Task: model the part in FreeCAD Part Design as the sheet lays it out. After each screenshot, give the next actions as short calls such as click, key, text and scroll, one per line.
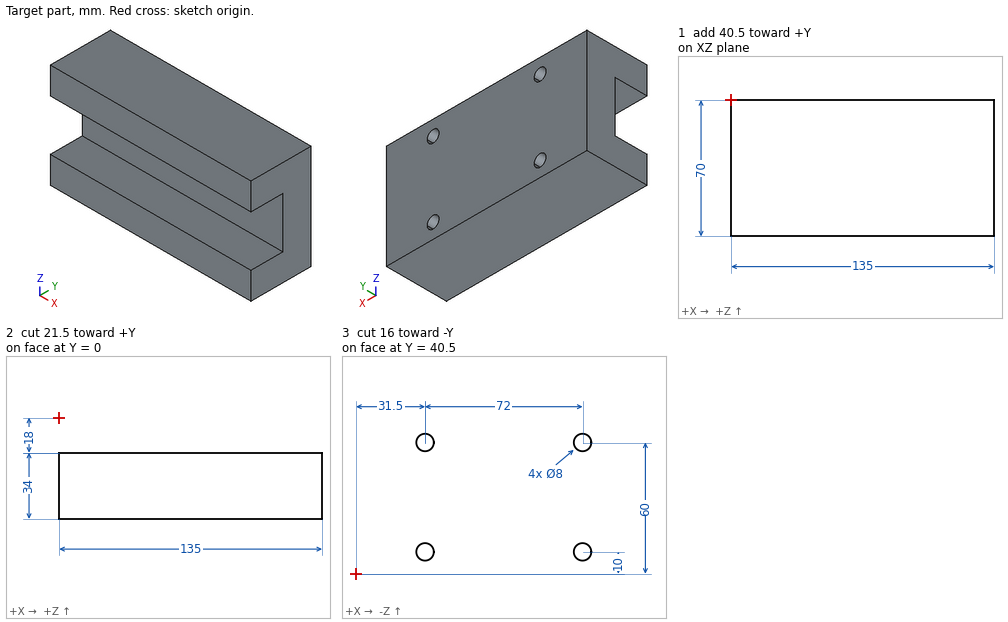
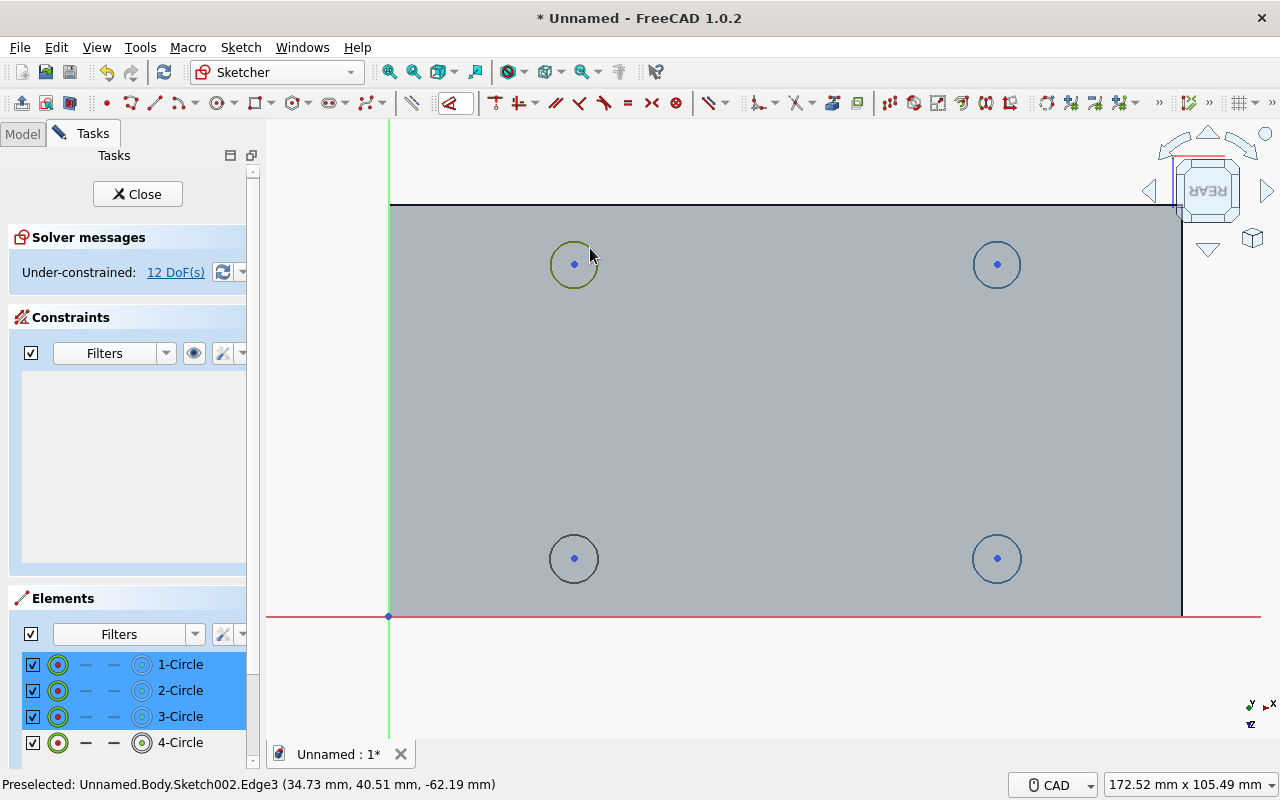
click(591, 542)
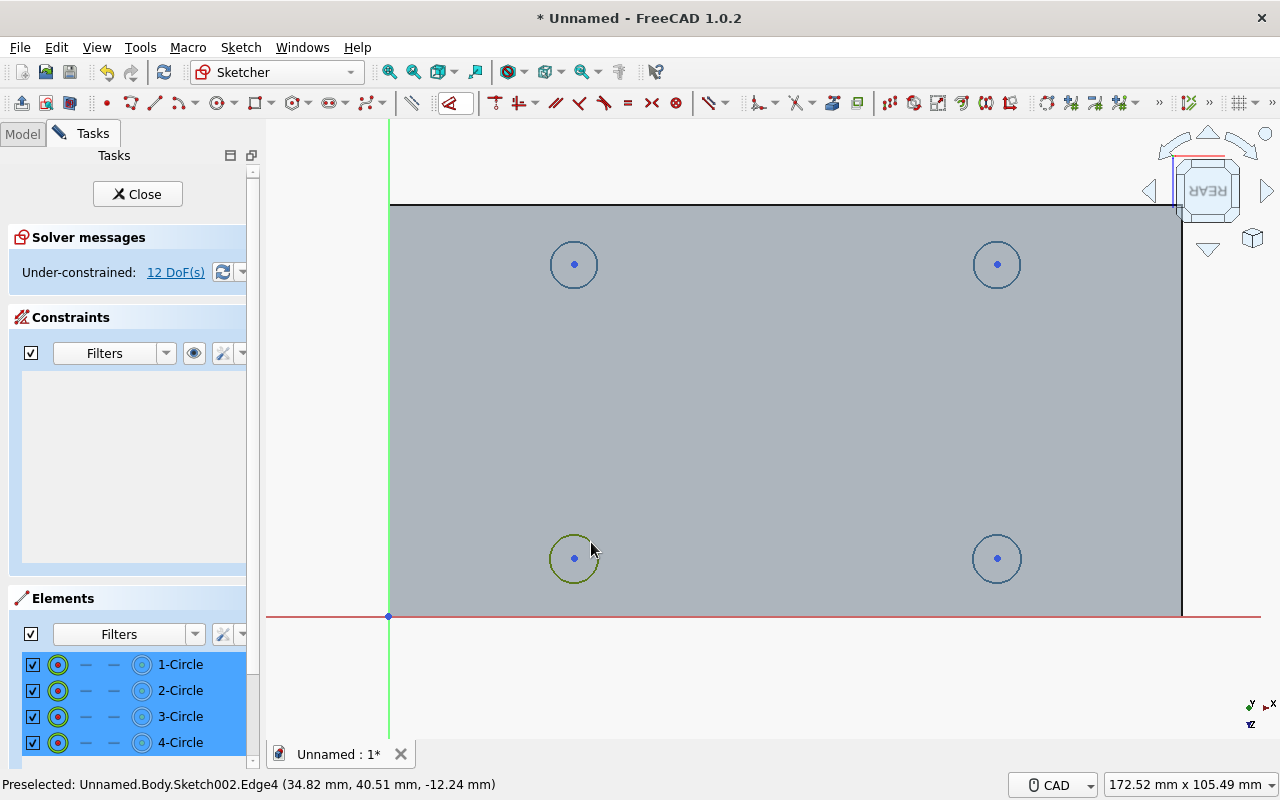
click(628, 104)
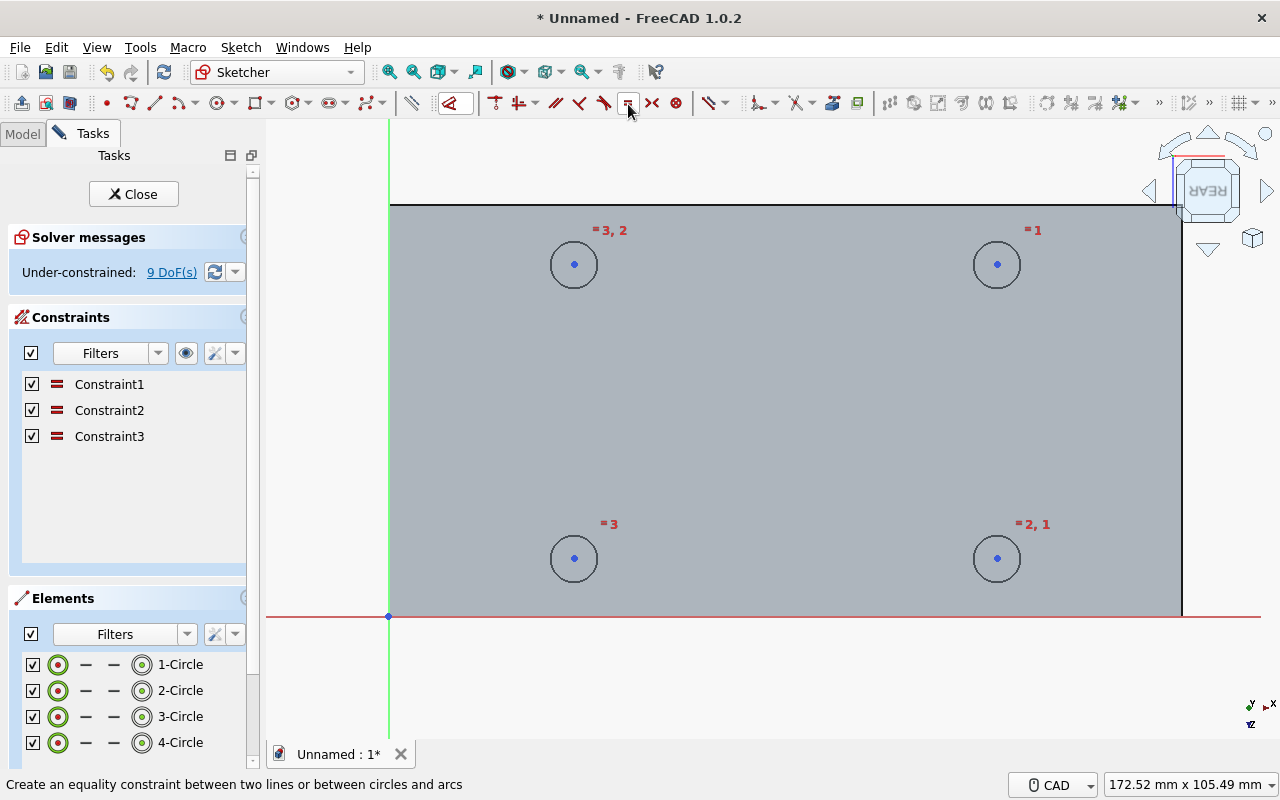
click(997, 265)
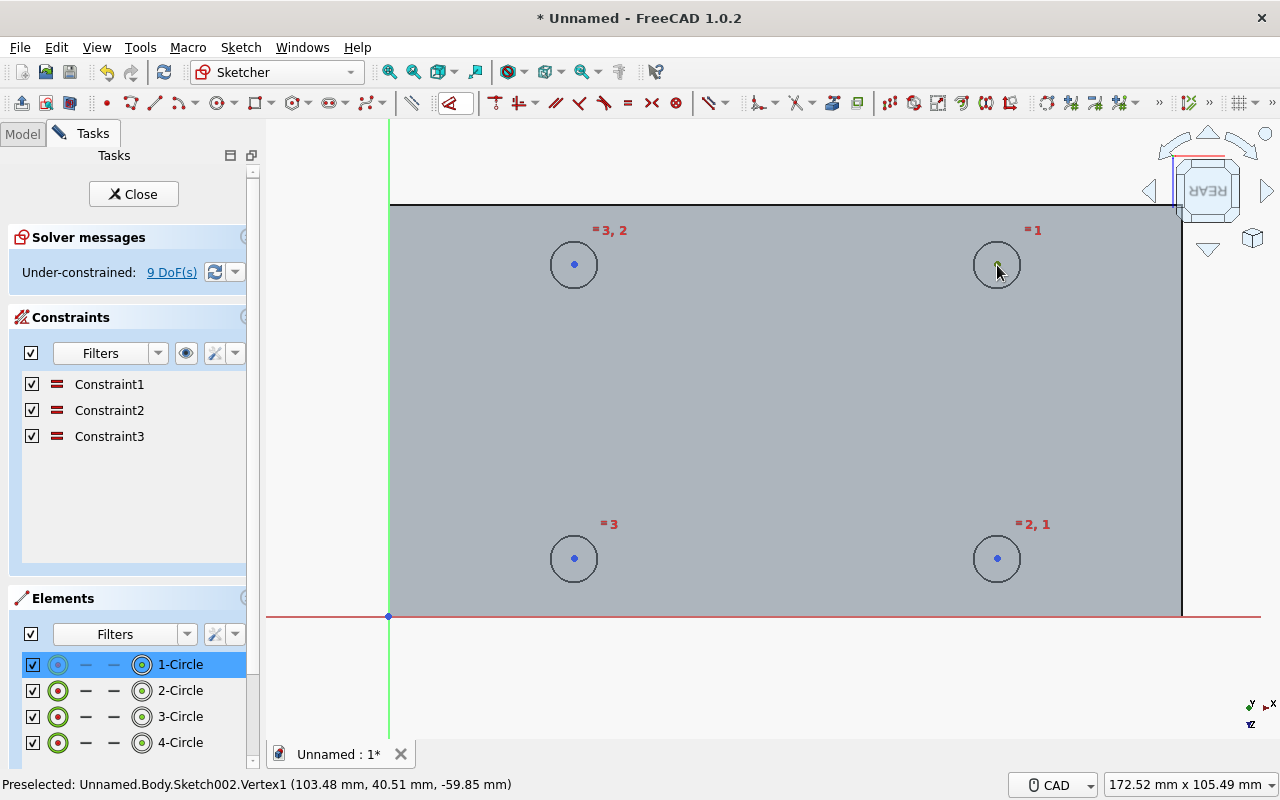
click(997, 559)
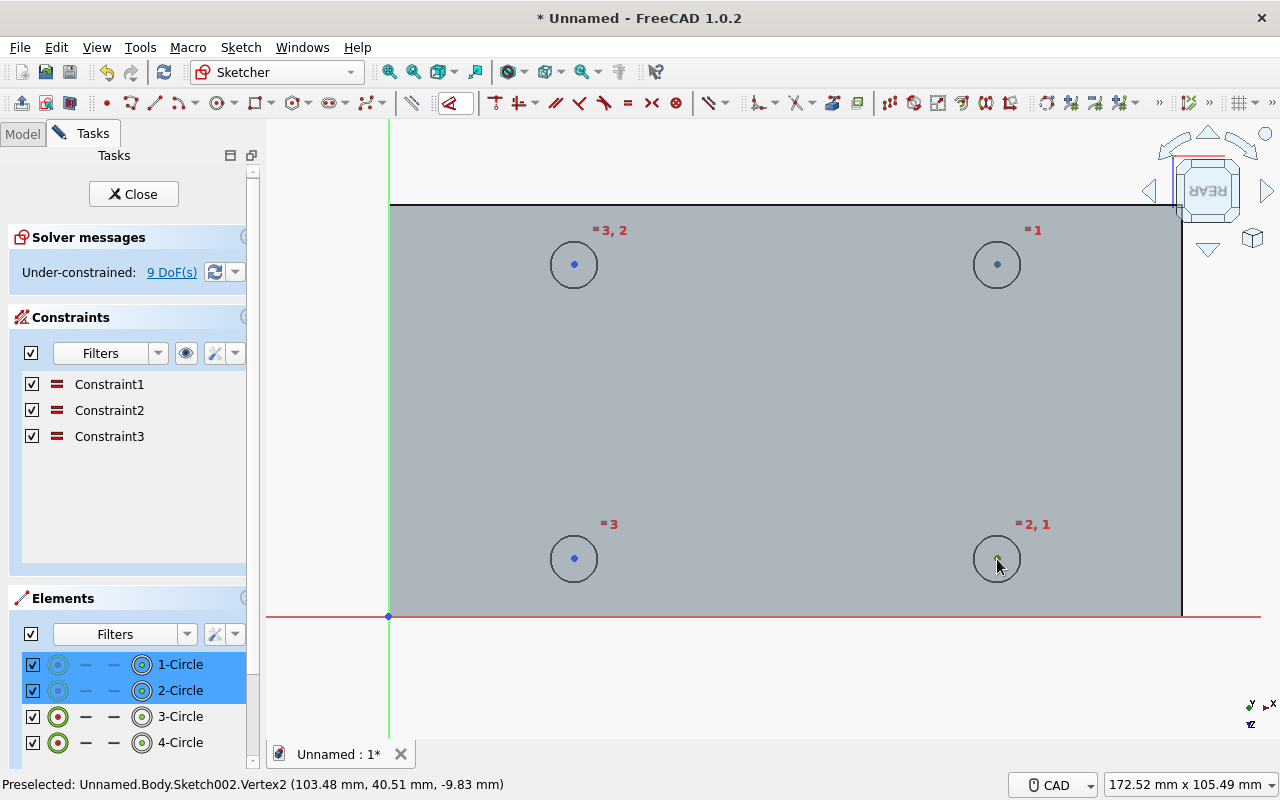
click(538, 104)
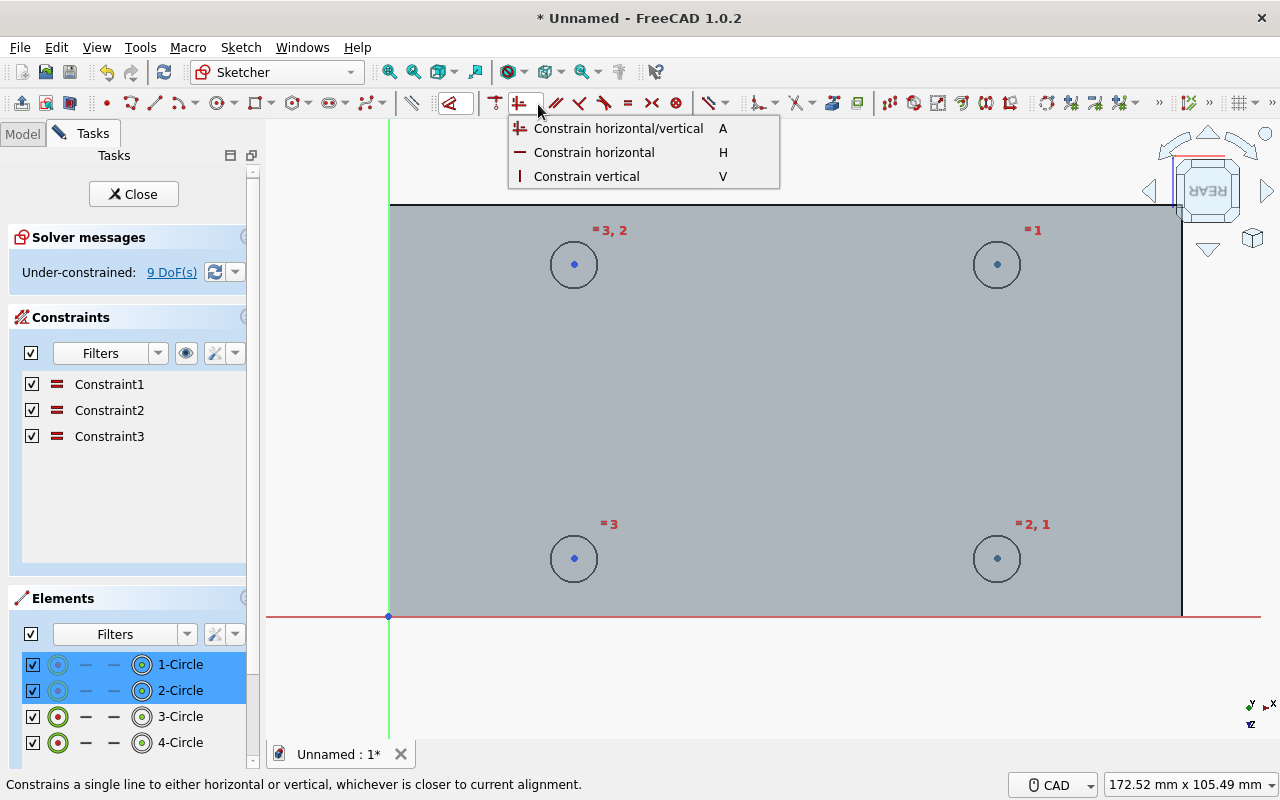
click(644, 176)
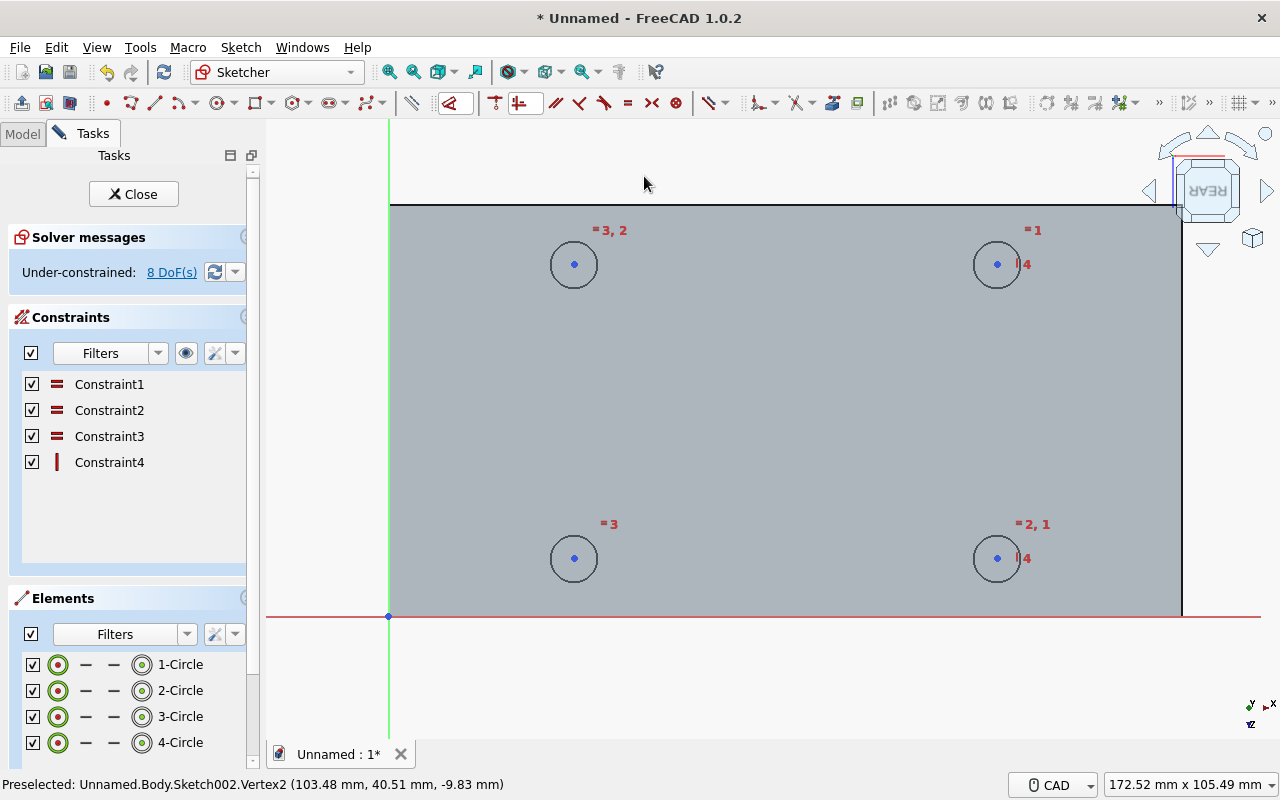
click(997, 265)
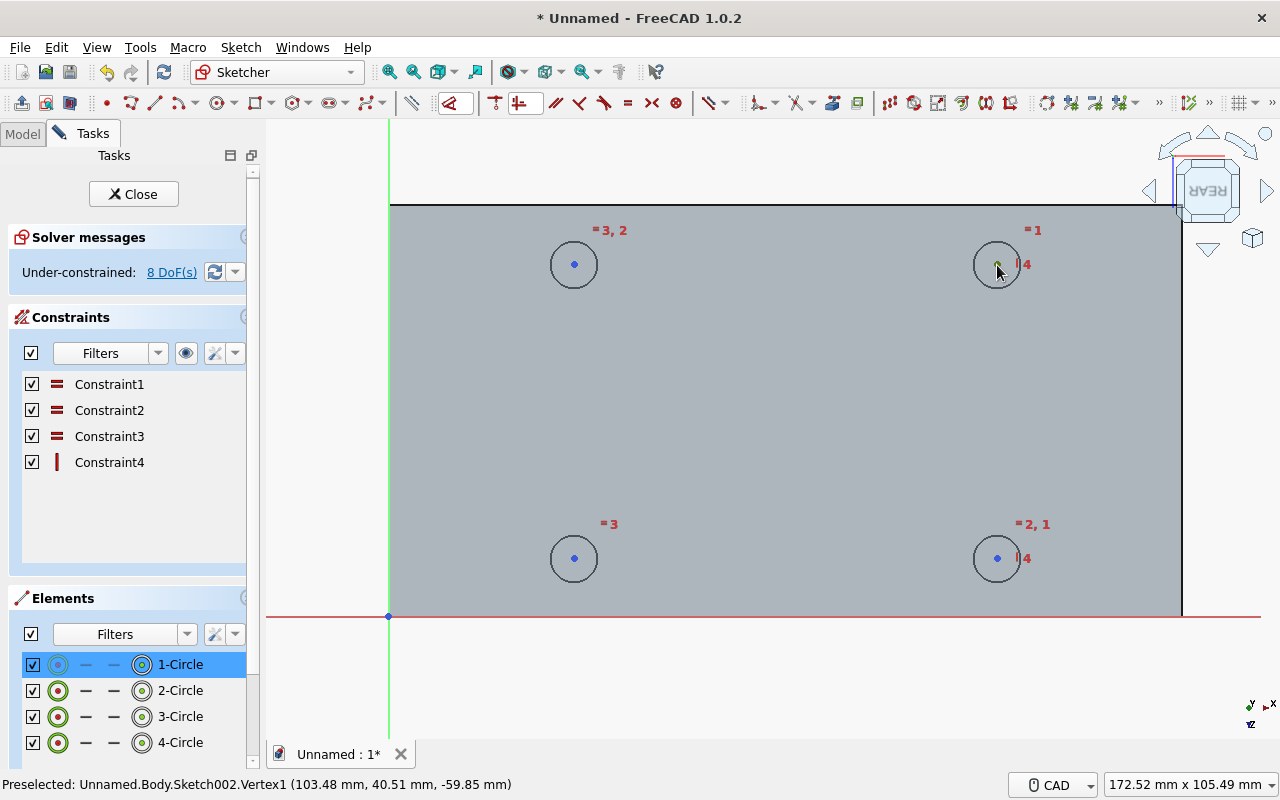
click(574, 265)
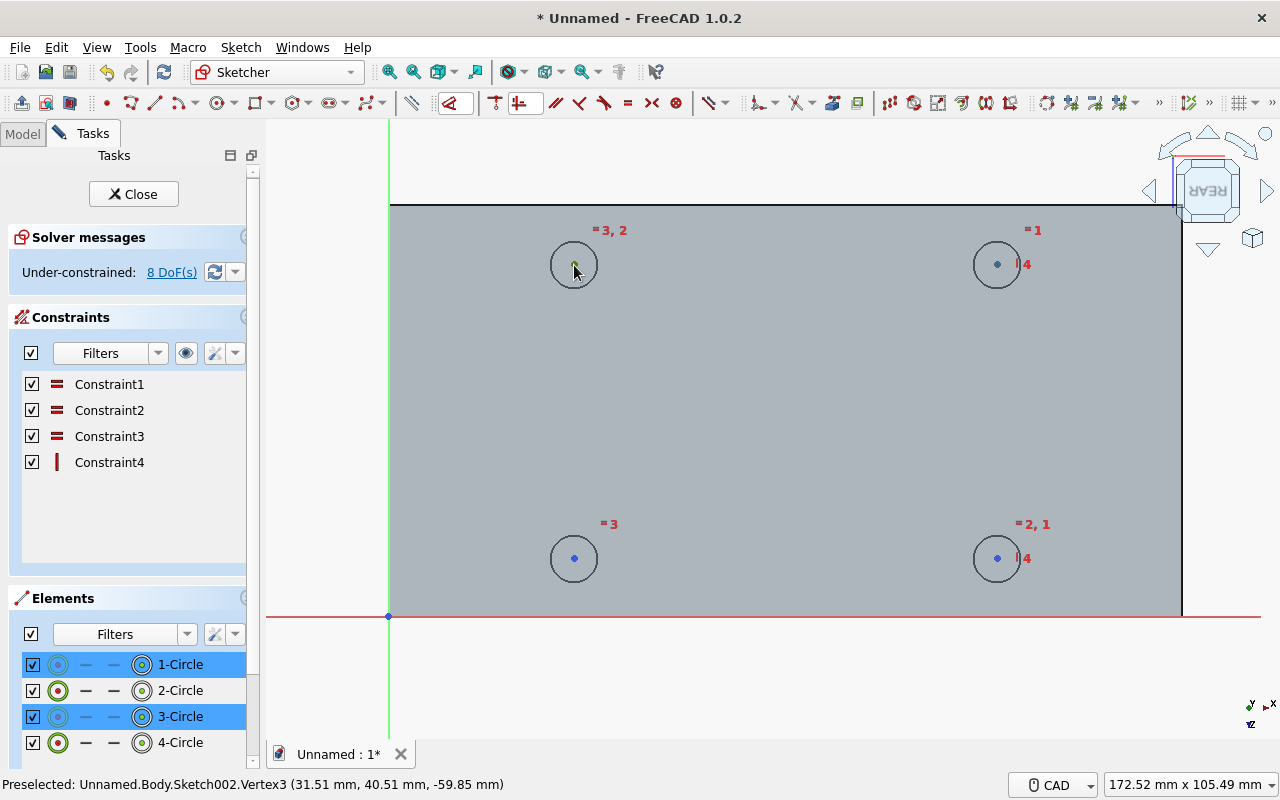
click(538, 104)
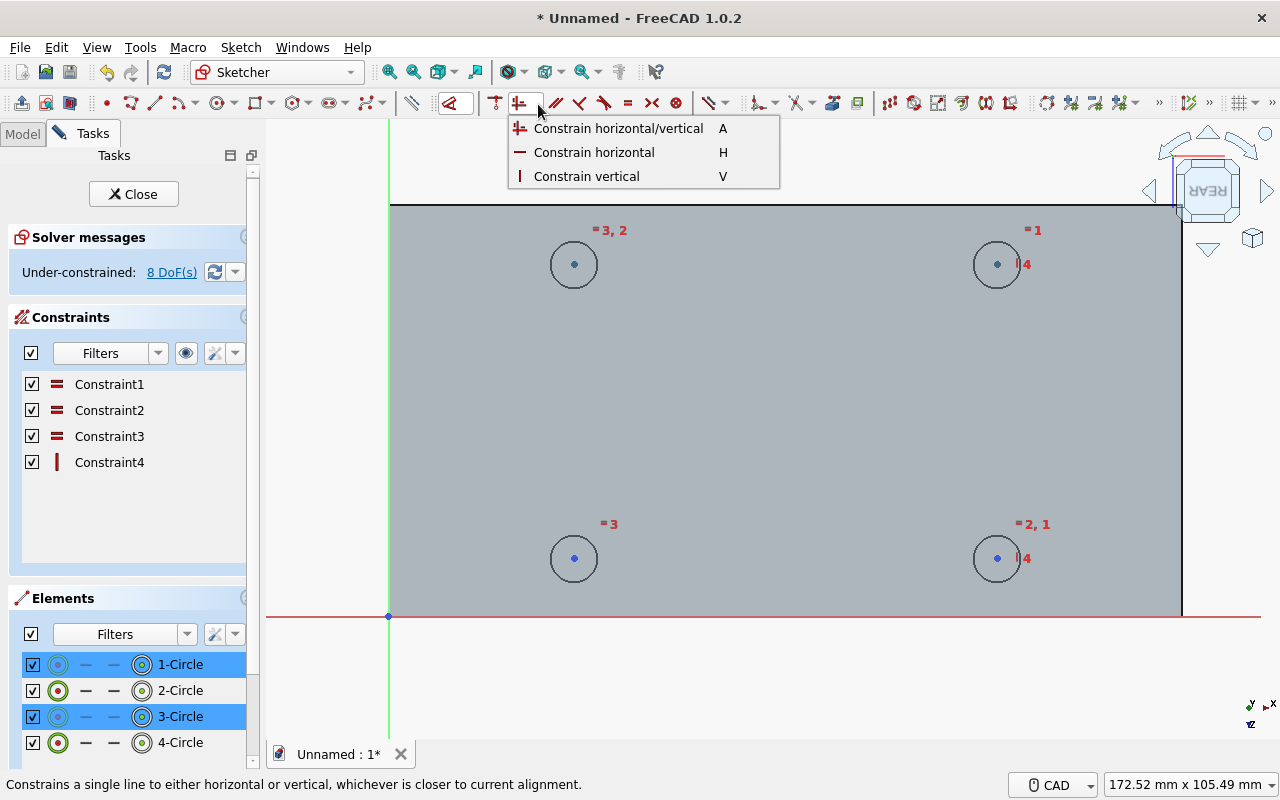
click(644, 152)